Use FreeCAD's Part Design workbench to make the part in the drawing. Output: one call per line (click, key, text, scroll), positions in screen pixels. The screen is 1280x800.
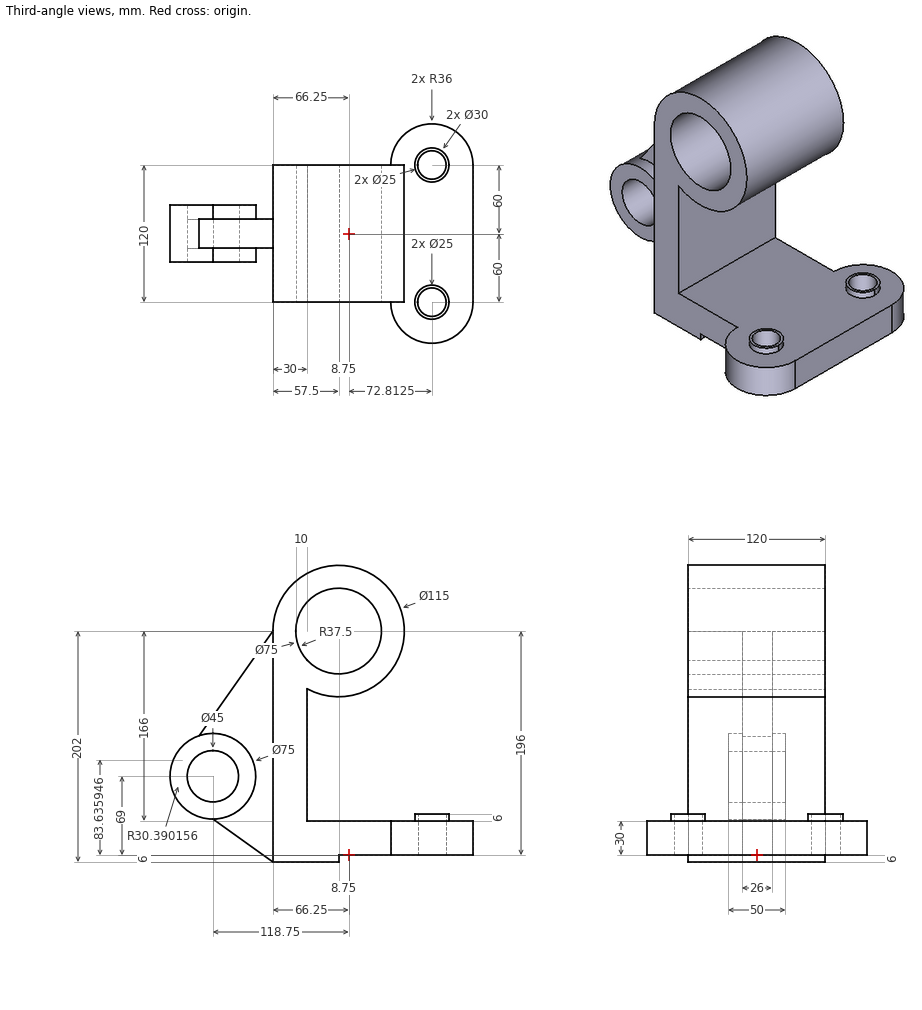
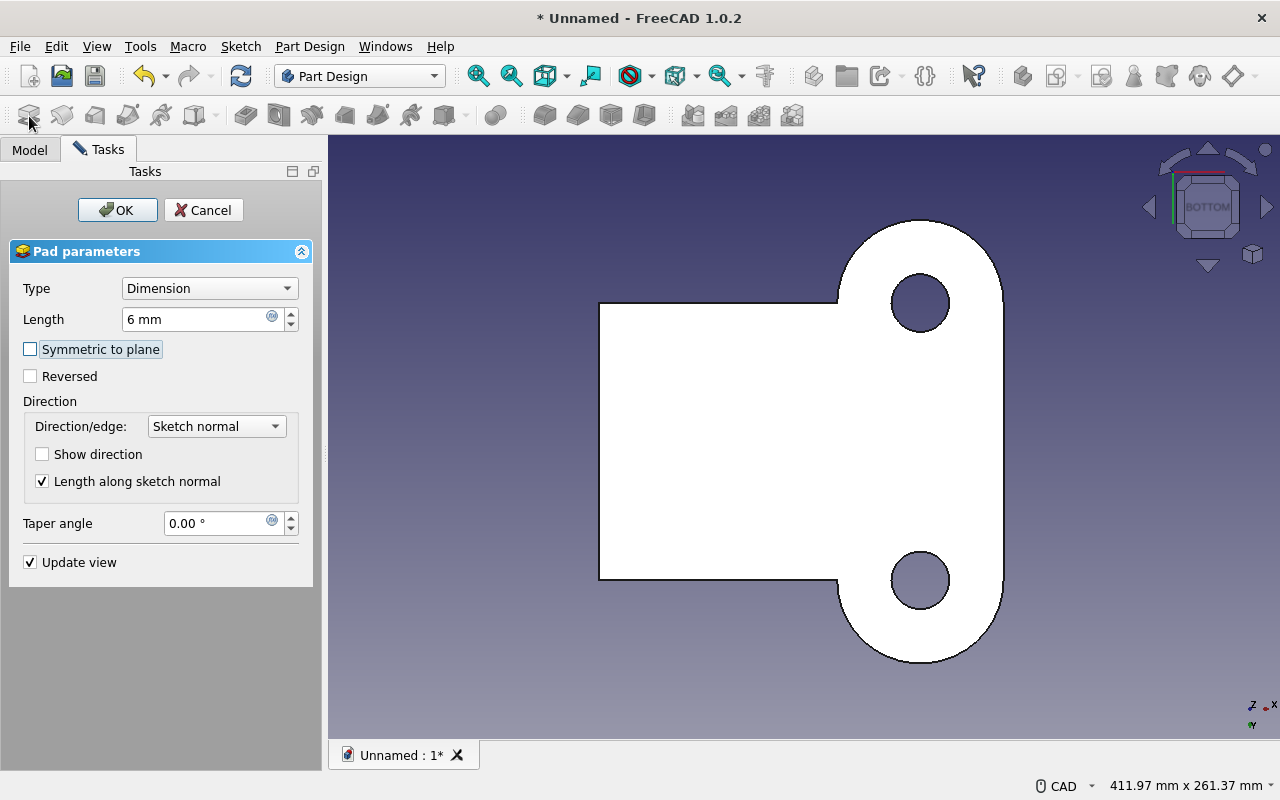
click(31, 376)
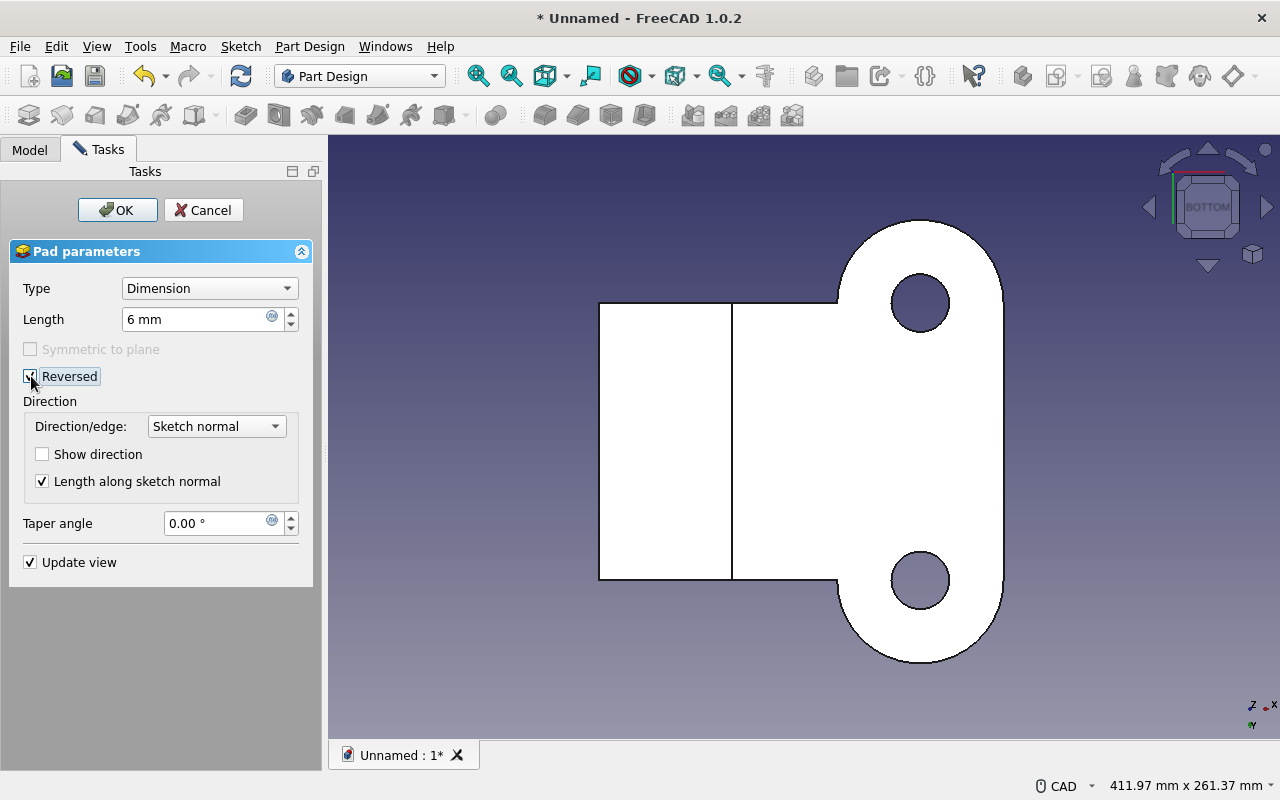
click(118, 210)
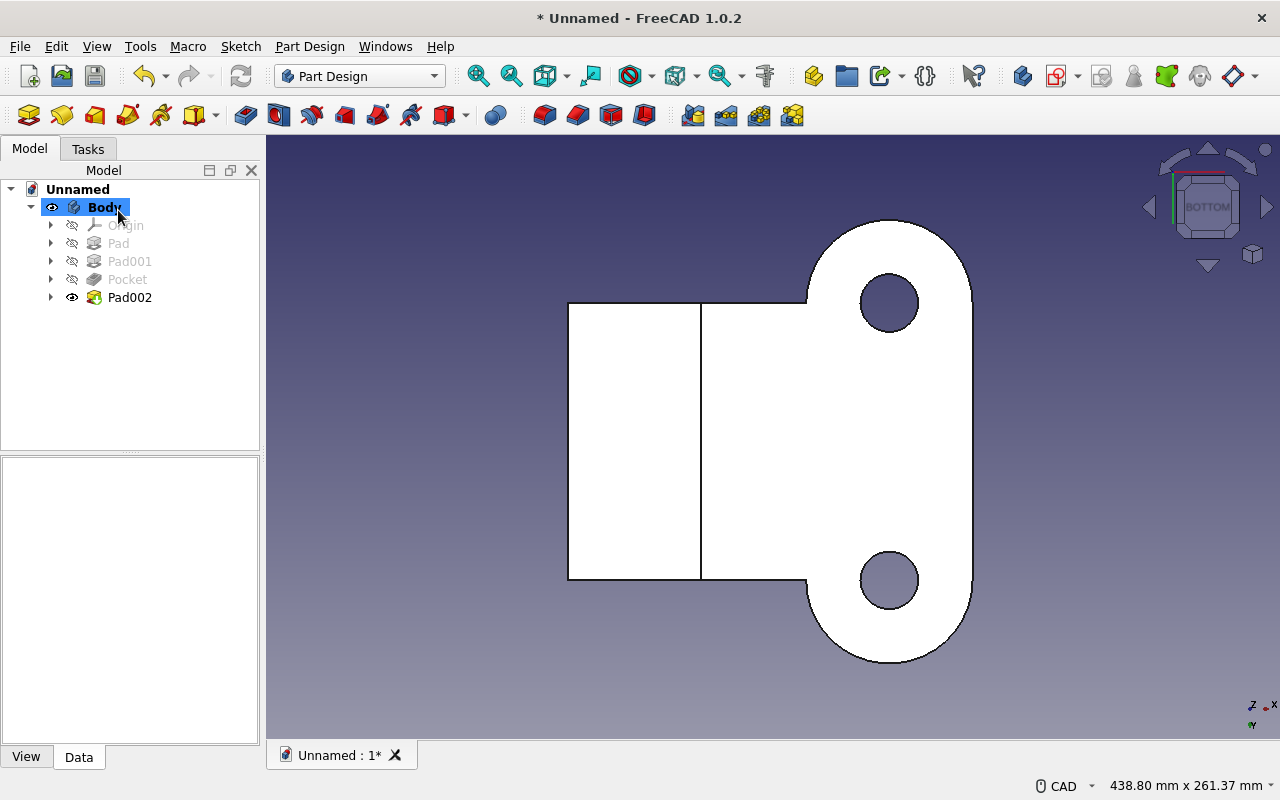
key(0)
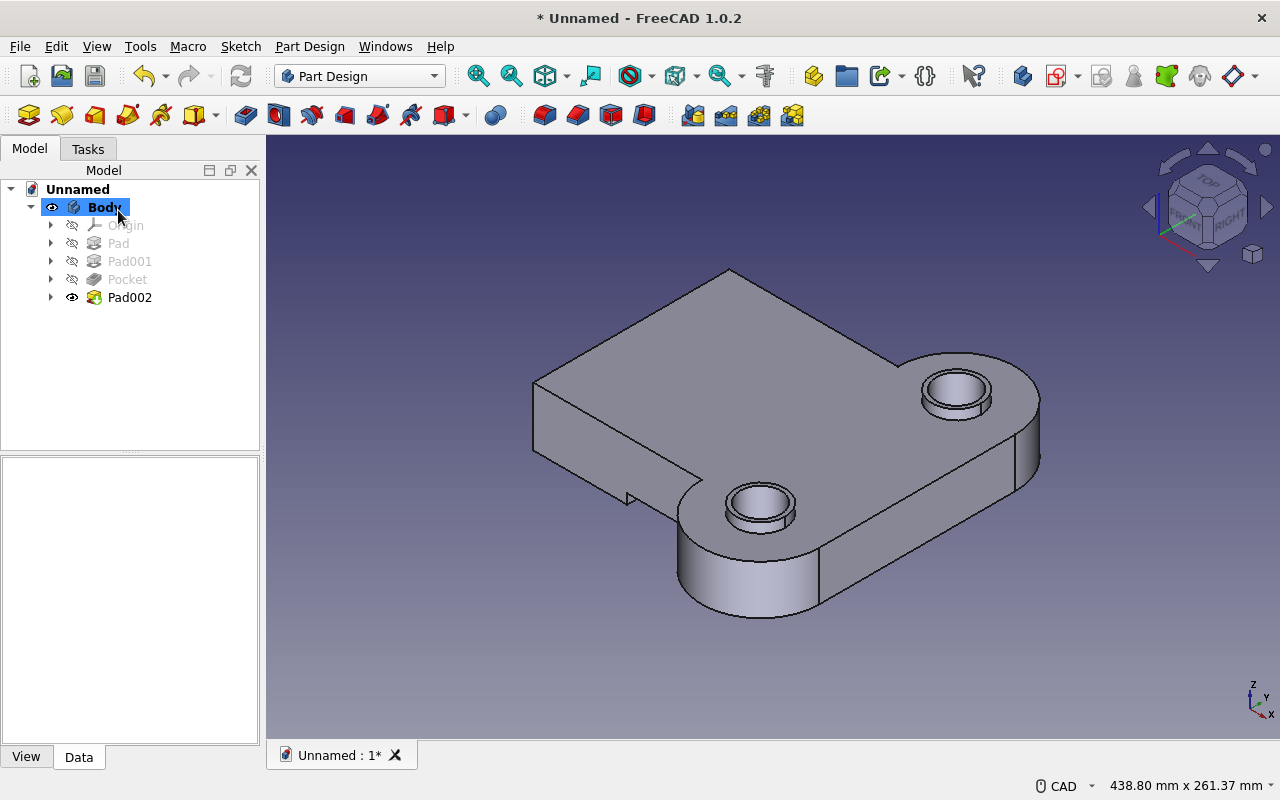
click(774, 408)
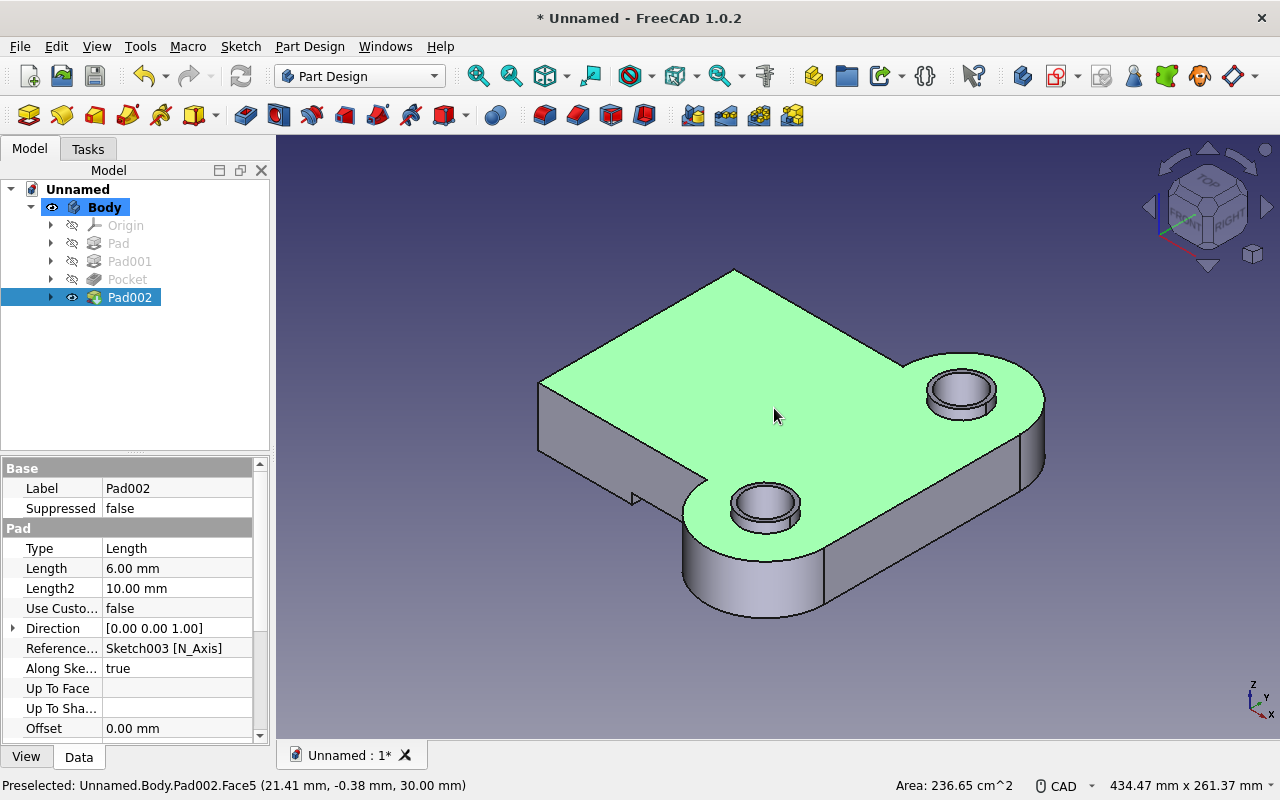
click(1056, 76)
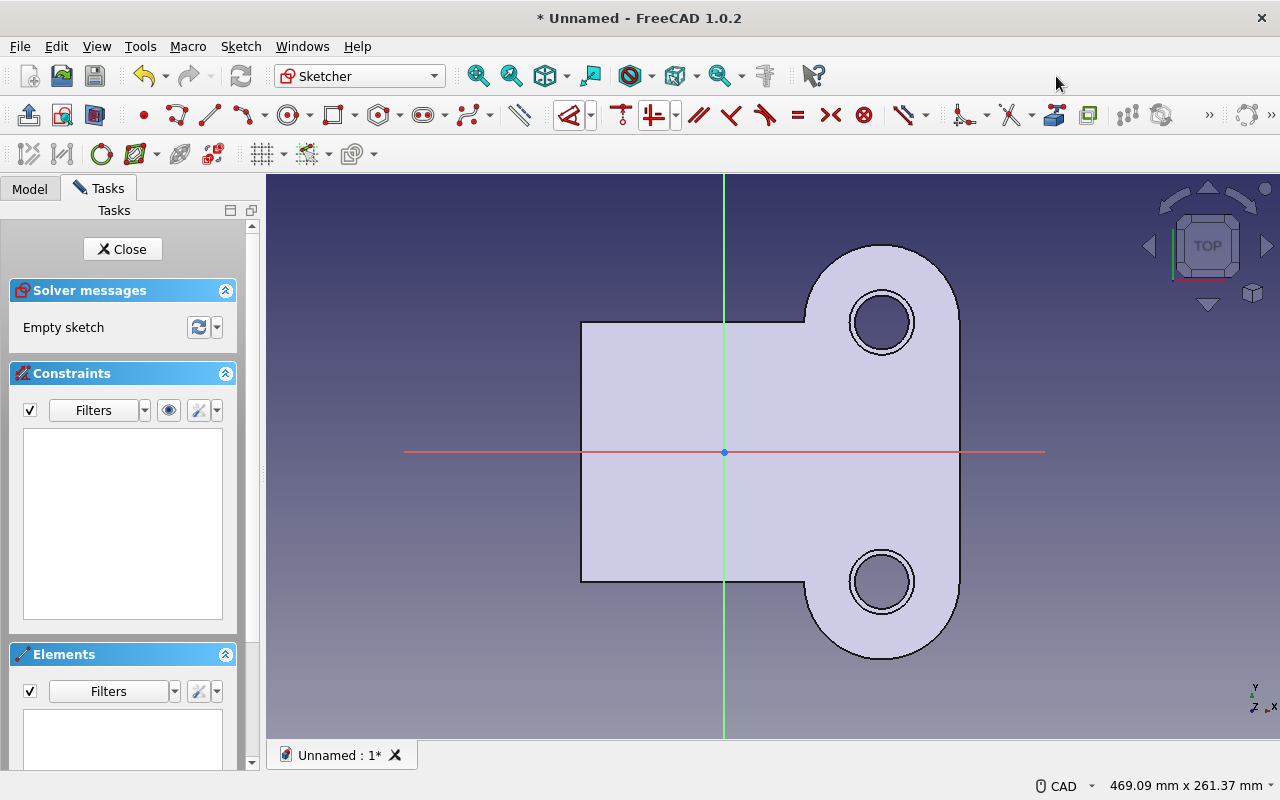
scroll(548, 443, up, 2)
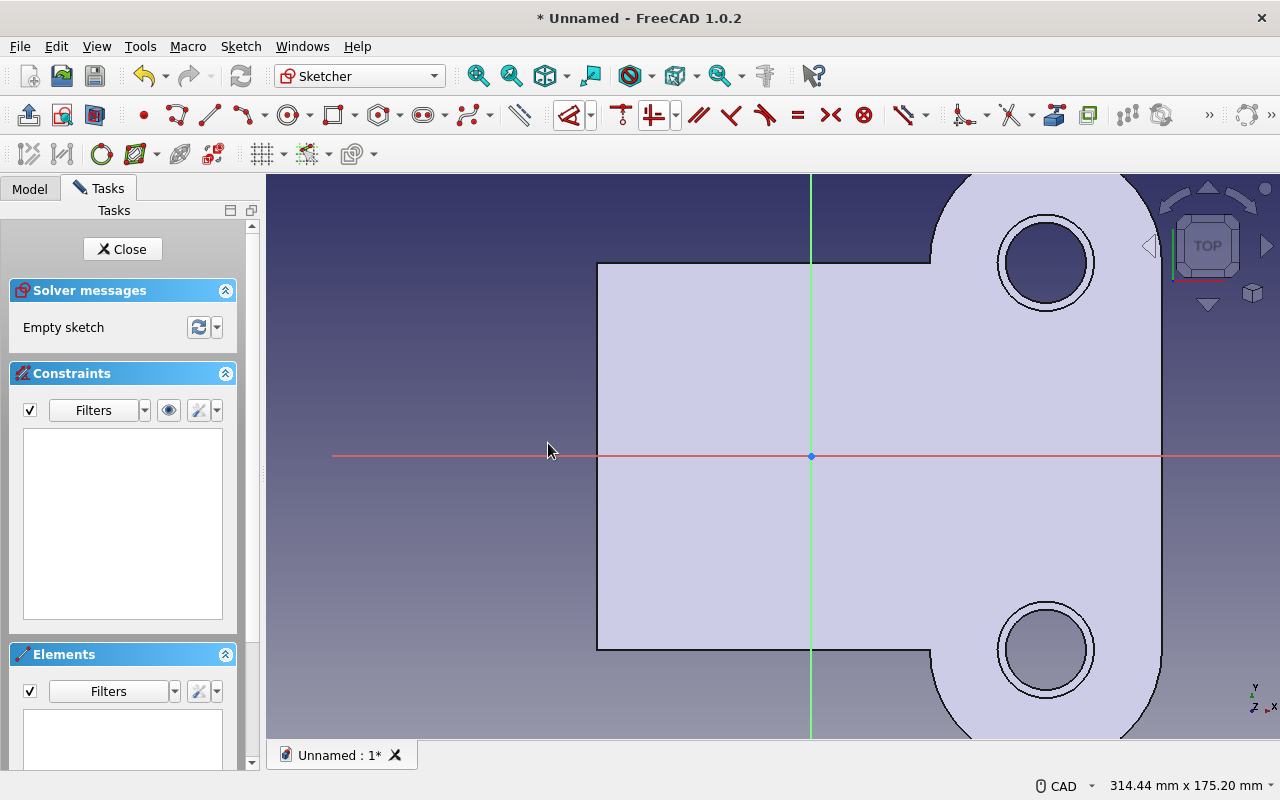
key(g)
key(r)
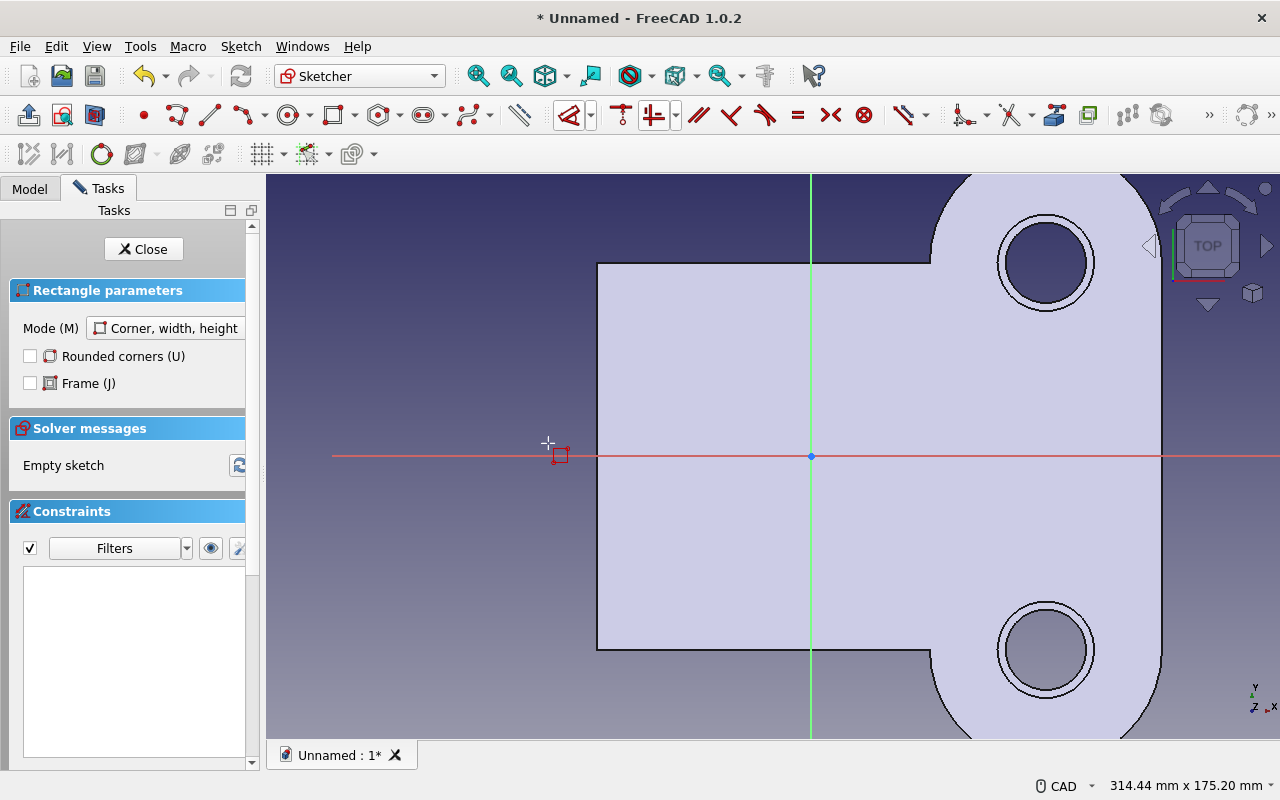
click(597, 263)
click(694, 650)
key(Escape)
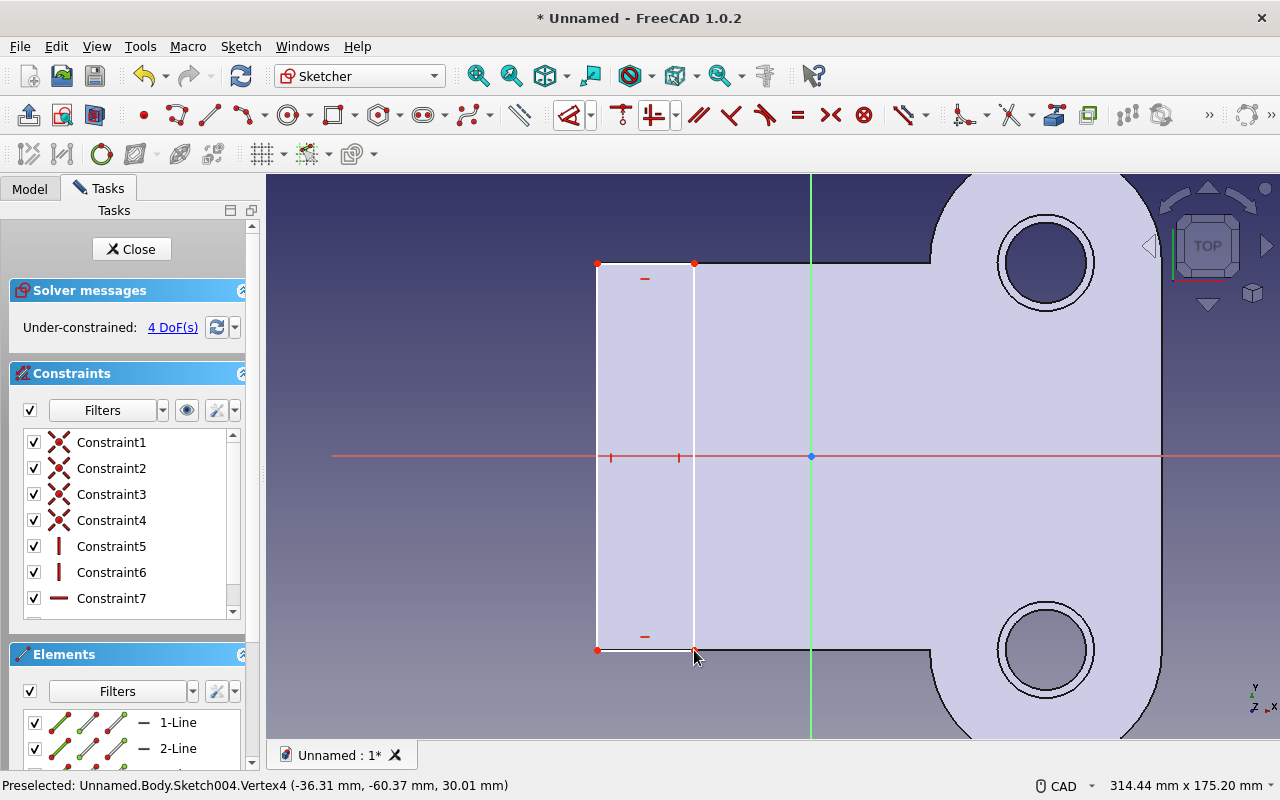
click(626, 651)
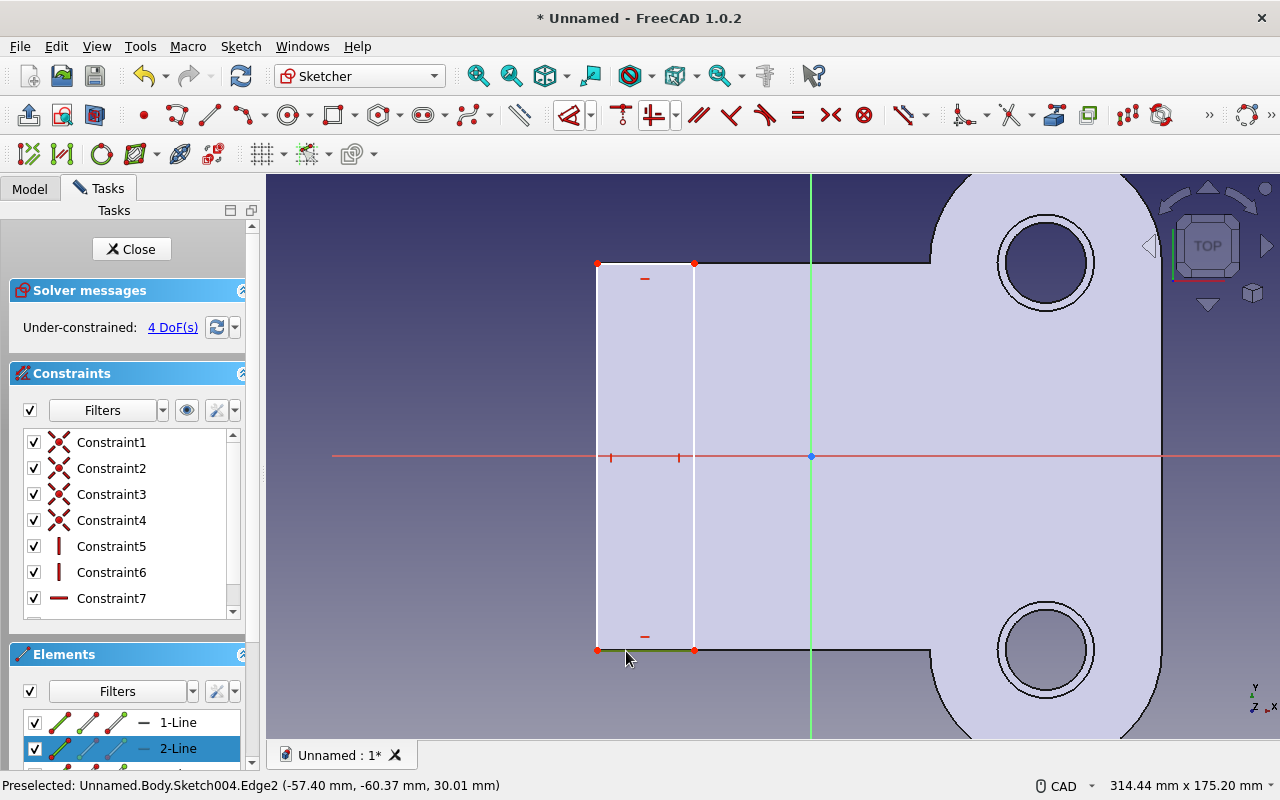
key(l)